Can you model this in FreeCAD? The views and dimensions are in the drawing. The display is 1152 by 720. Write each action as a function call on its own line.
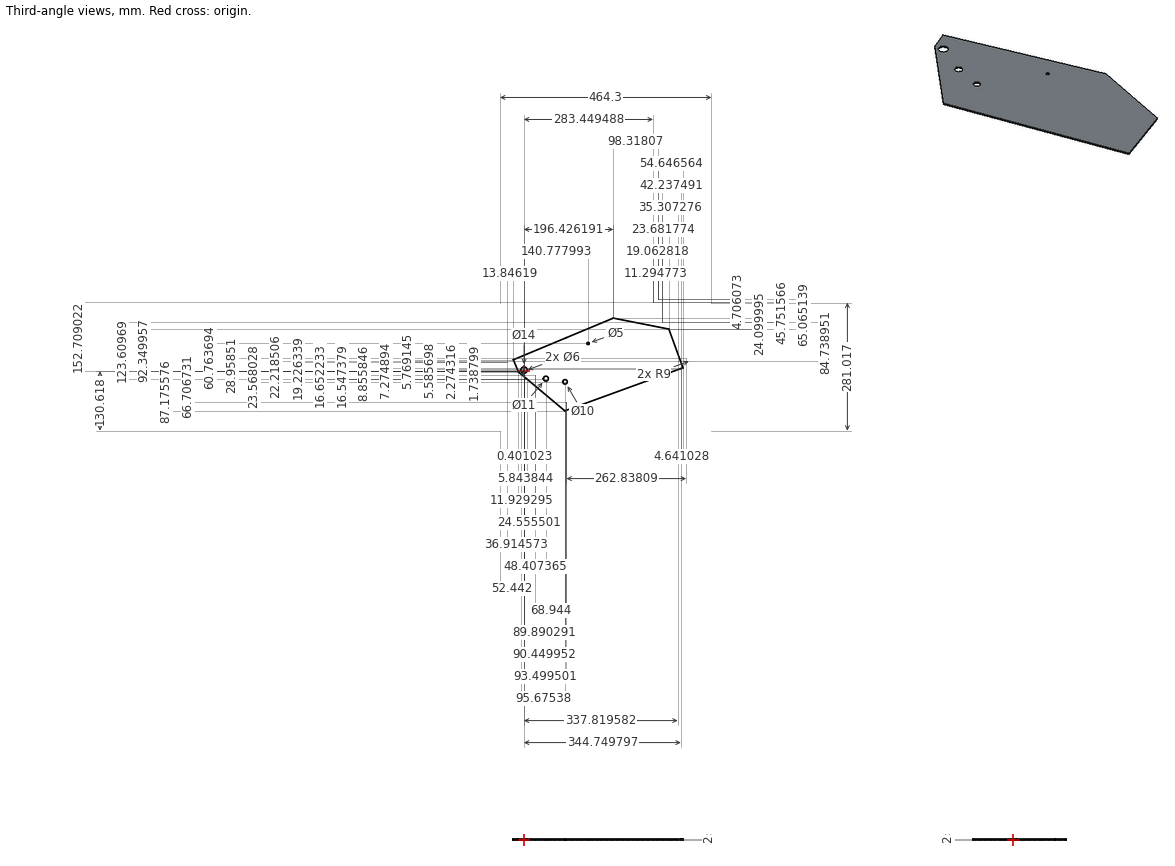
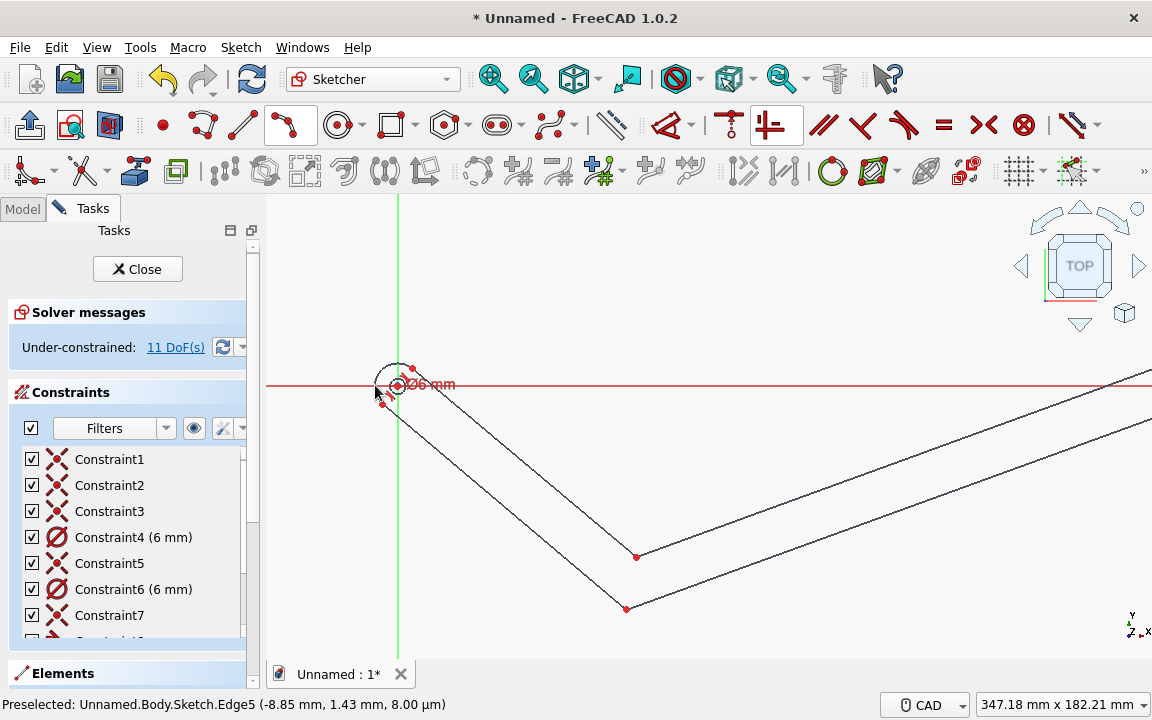
click(835, 534)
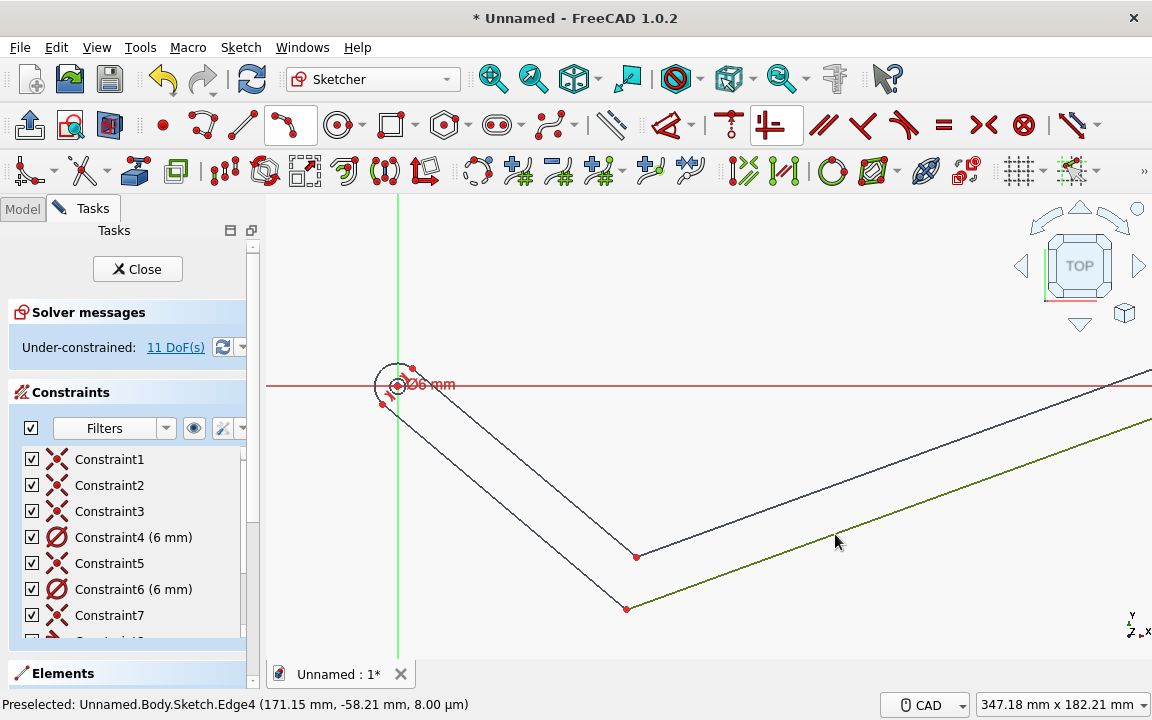
scroll(375, 386, down, 3)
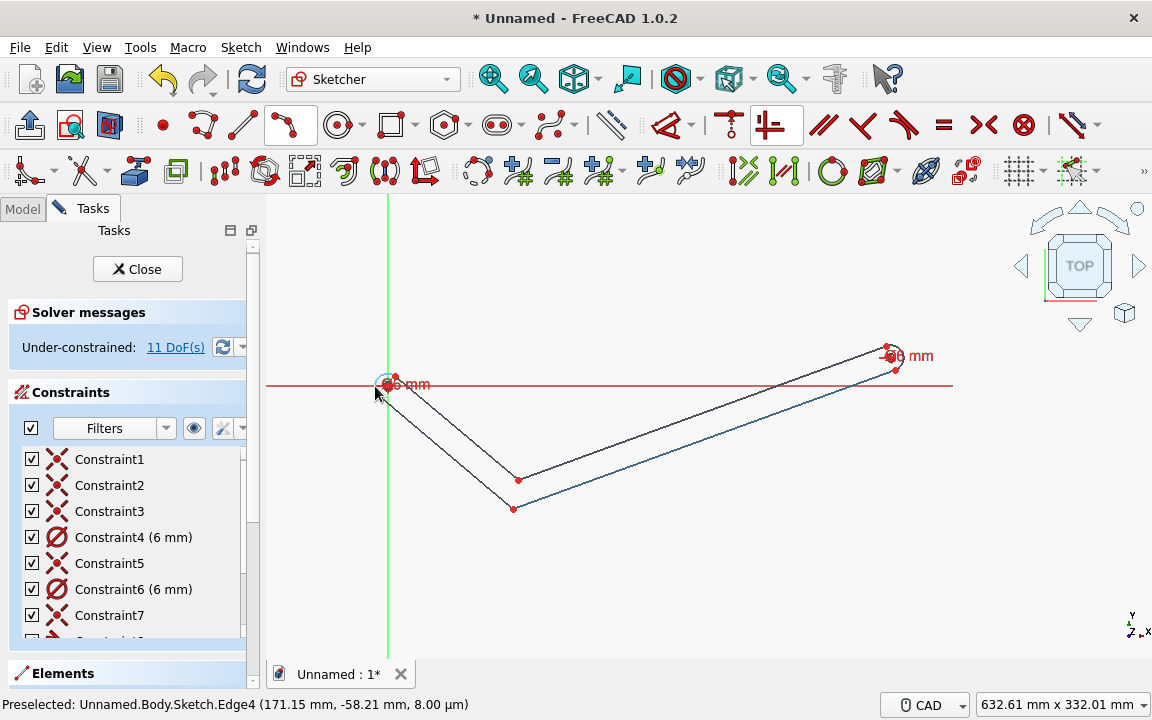
scroll(903, 362, up, 3)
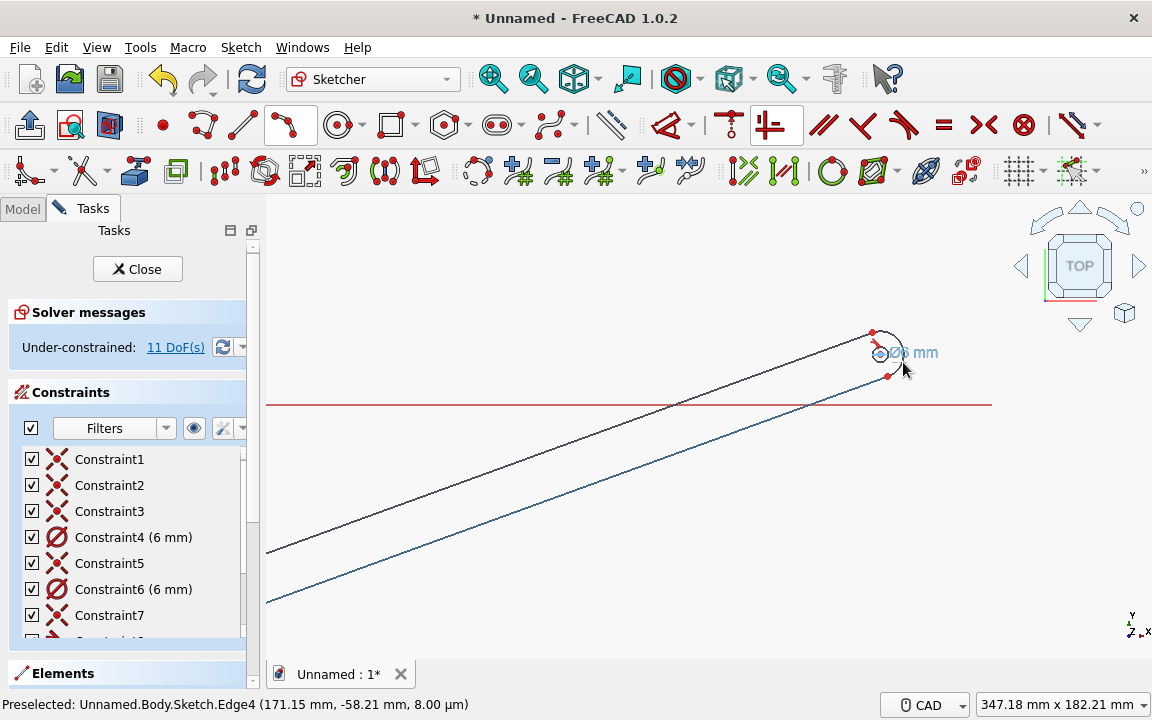
click(903, 361)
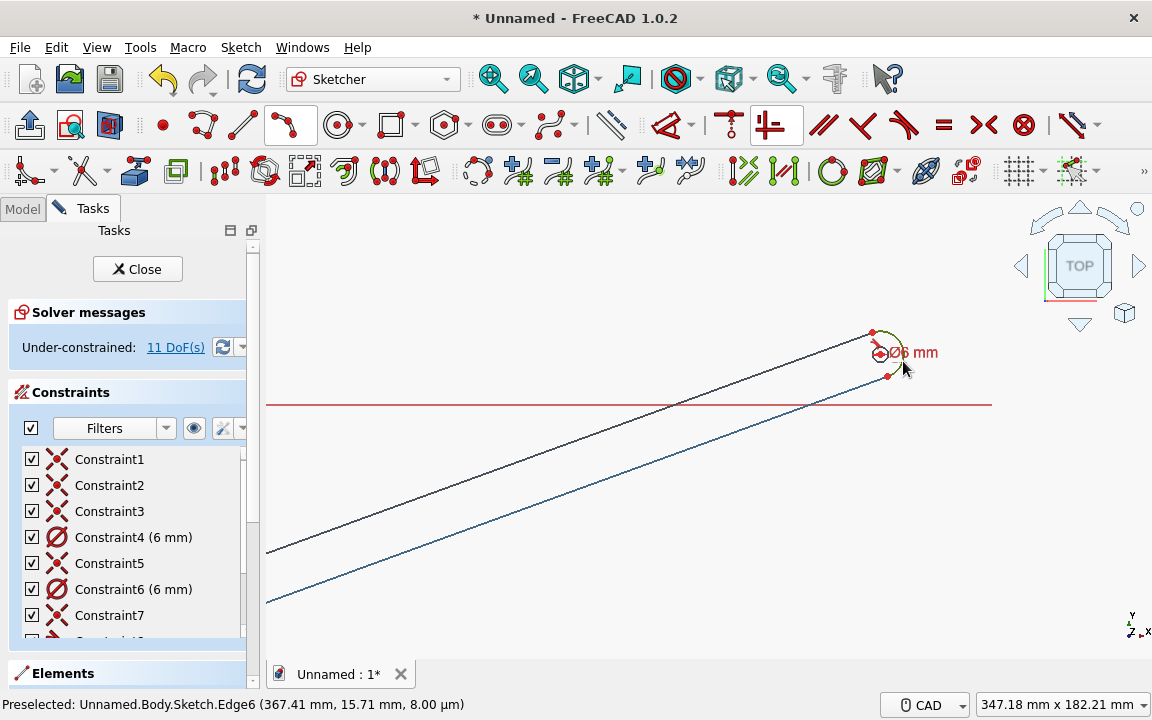
key(t)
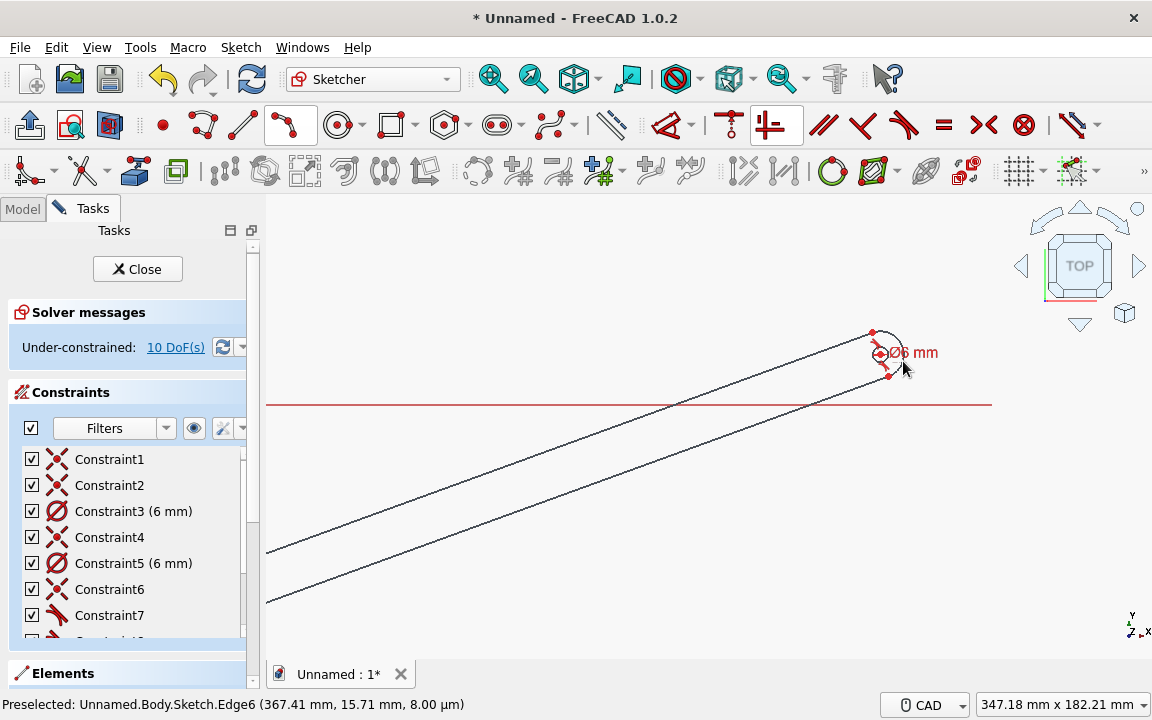
scroll(904, 362, down, 3)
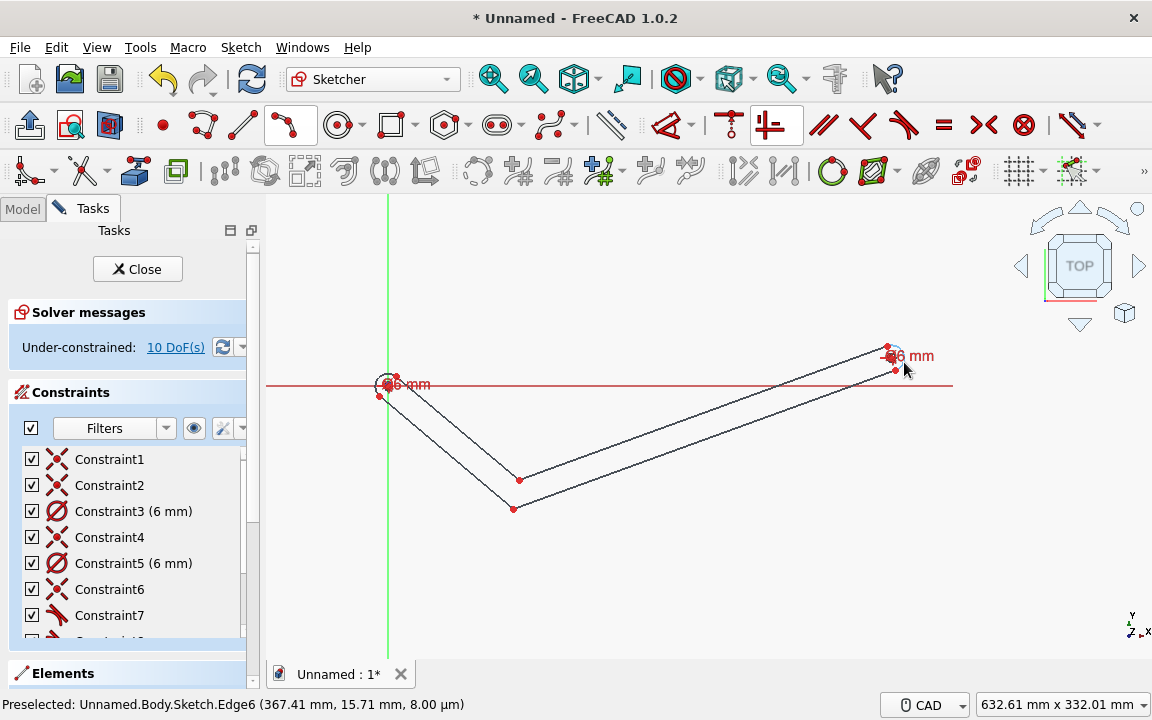
scroll(388, 386, up, 12)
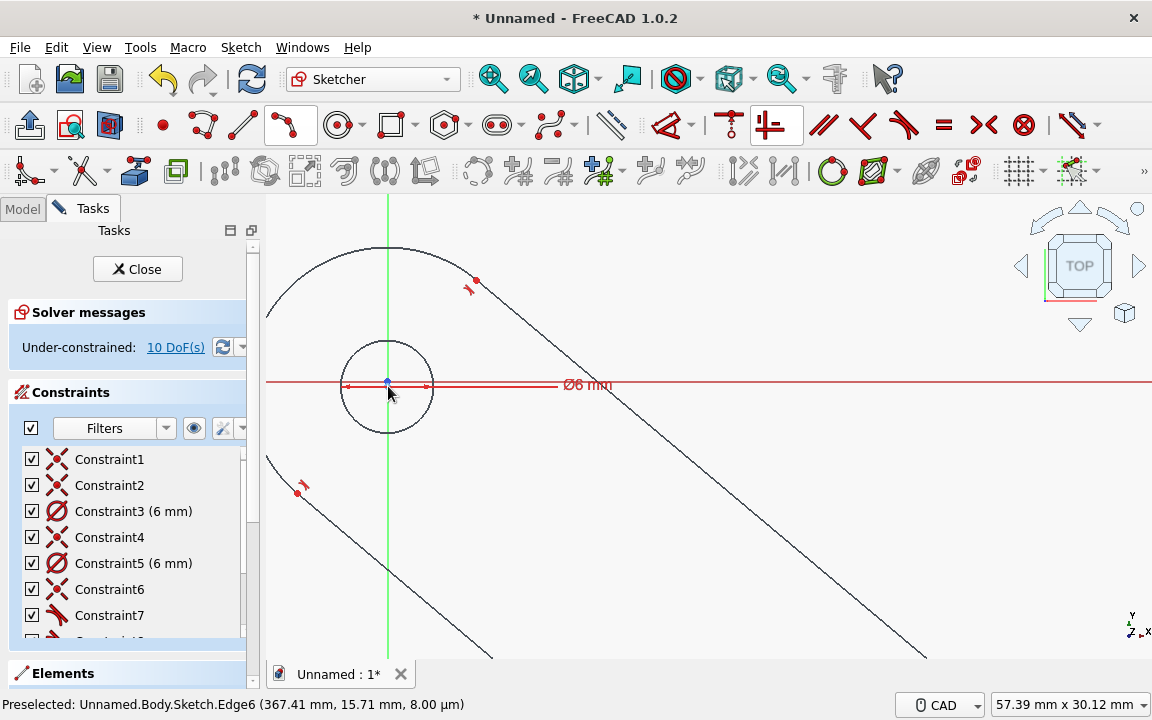
drag(377, 372, 398, 397)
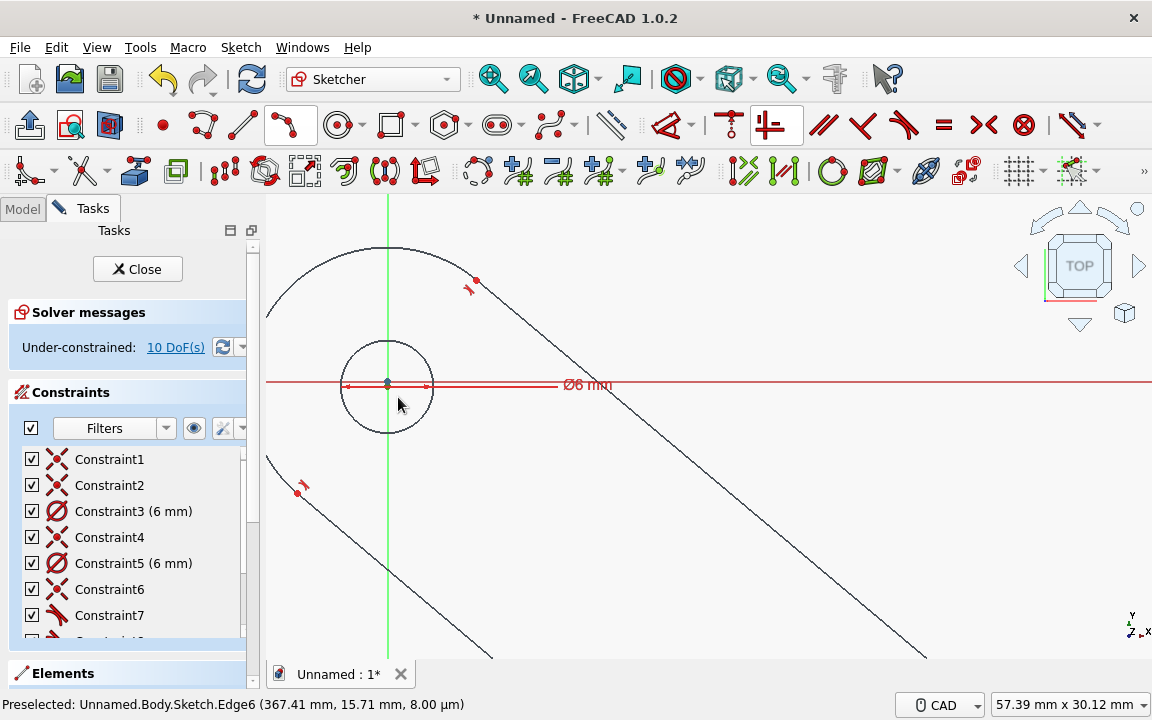
key(c)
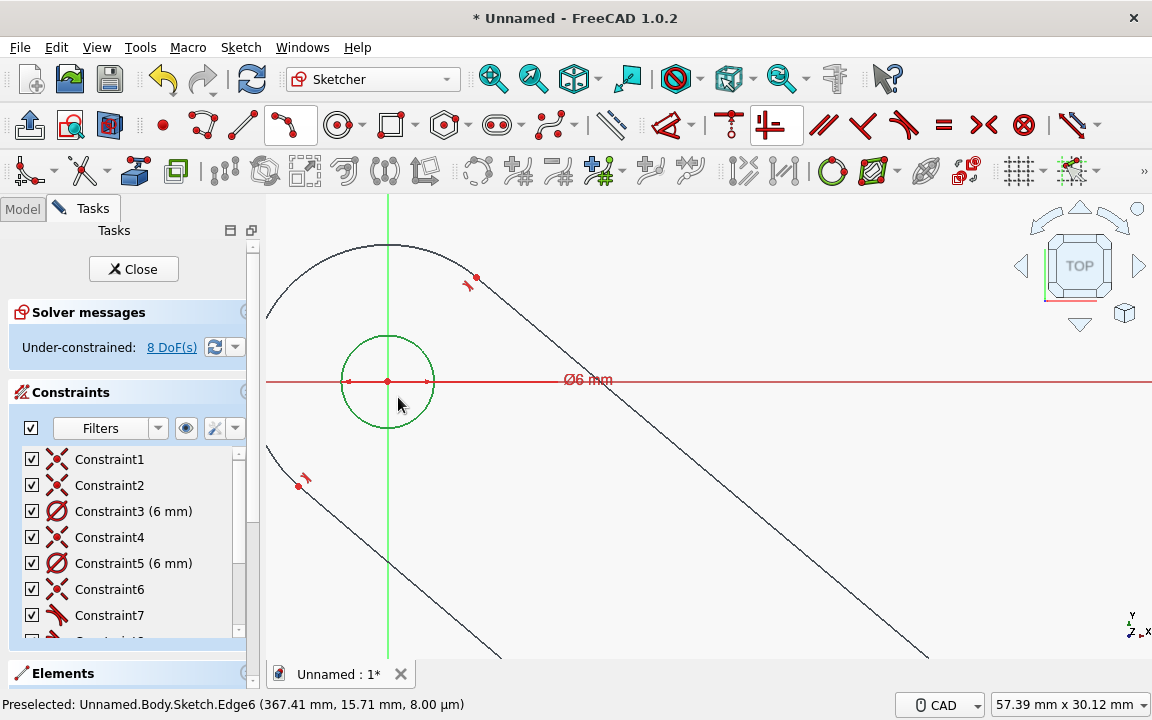
click(355, 249)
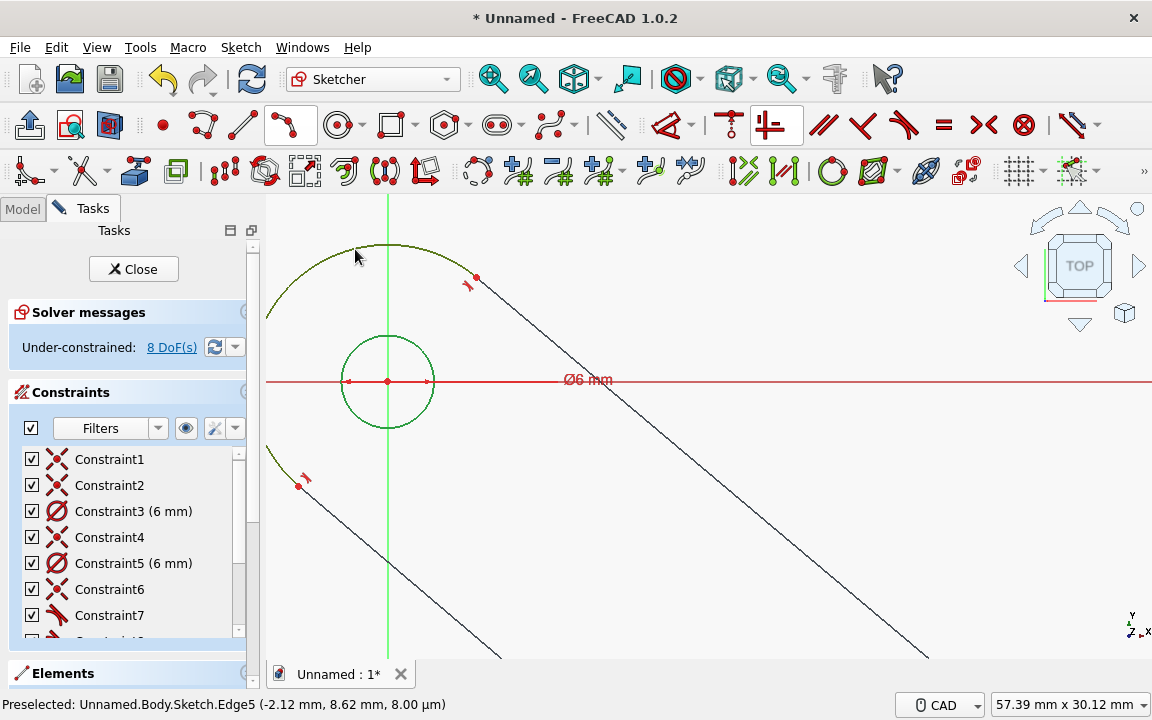
scroll(388, 386, down, 12)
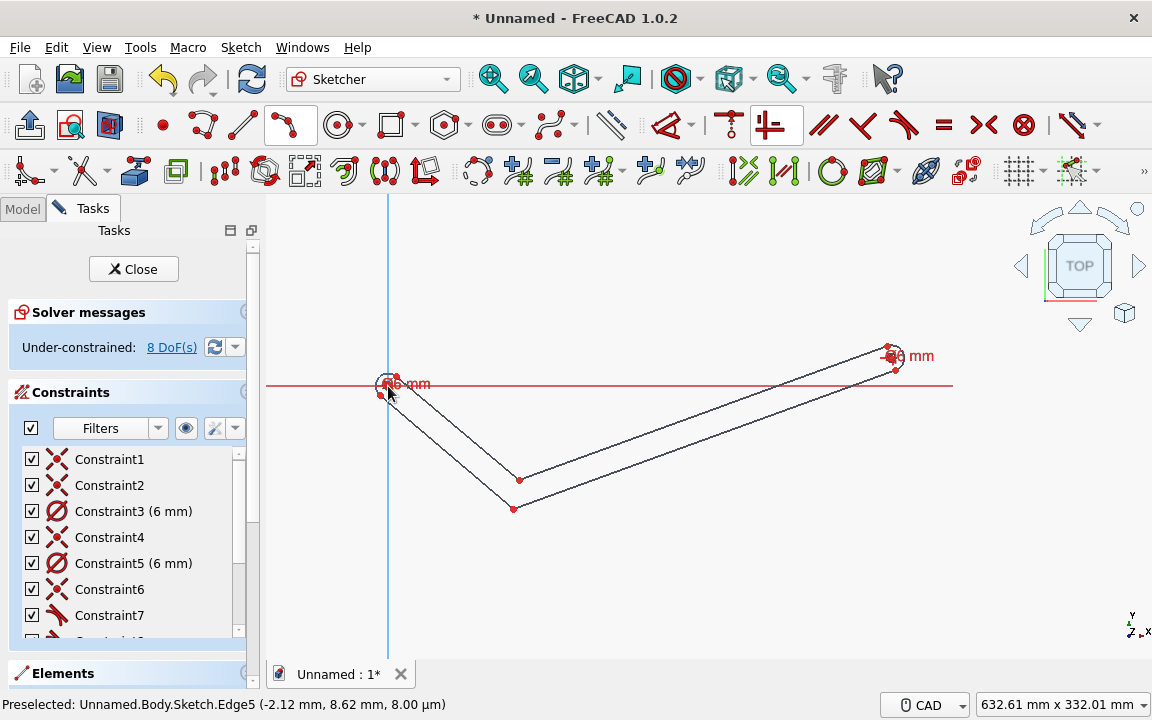
scroll(904, 362, up, 3)